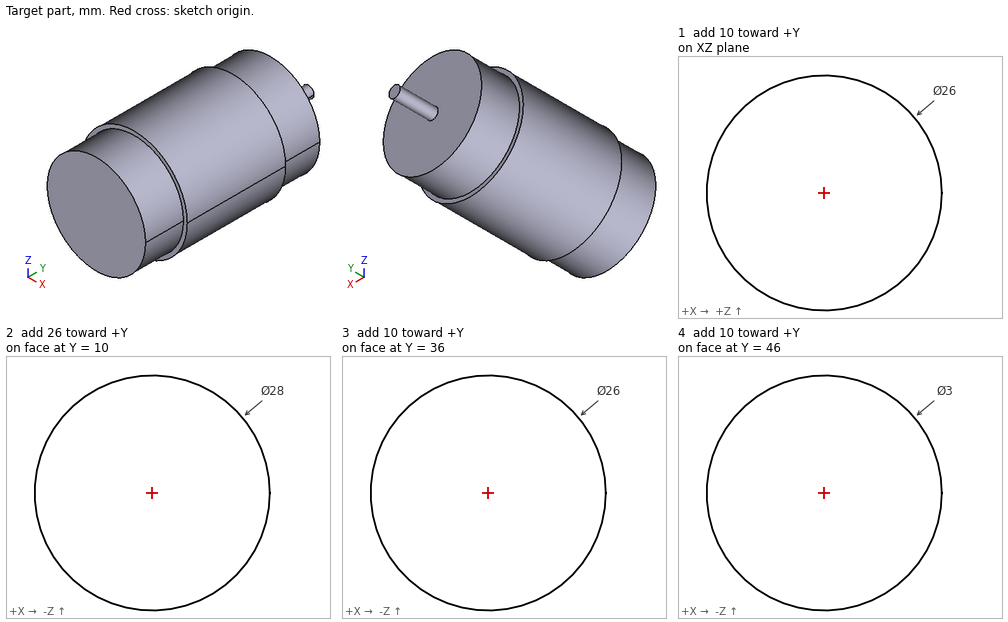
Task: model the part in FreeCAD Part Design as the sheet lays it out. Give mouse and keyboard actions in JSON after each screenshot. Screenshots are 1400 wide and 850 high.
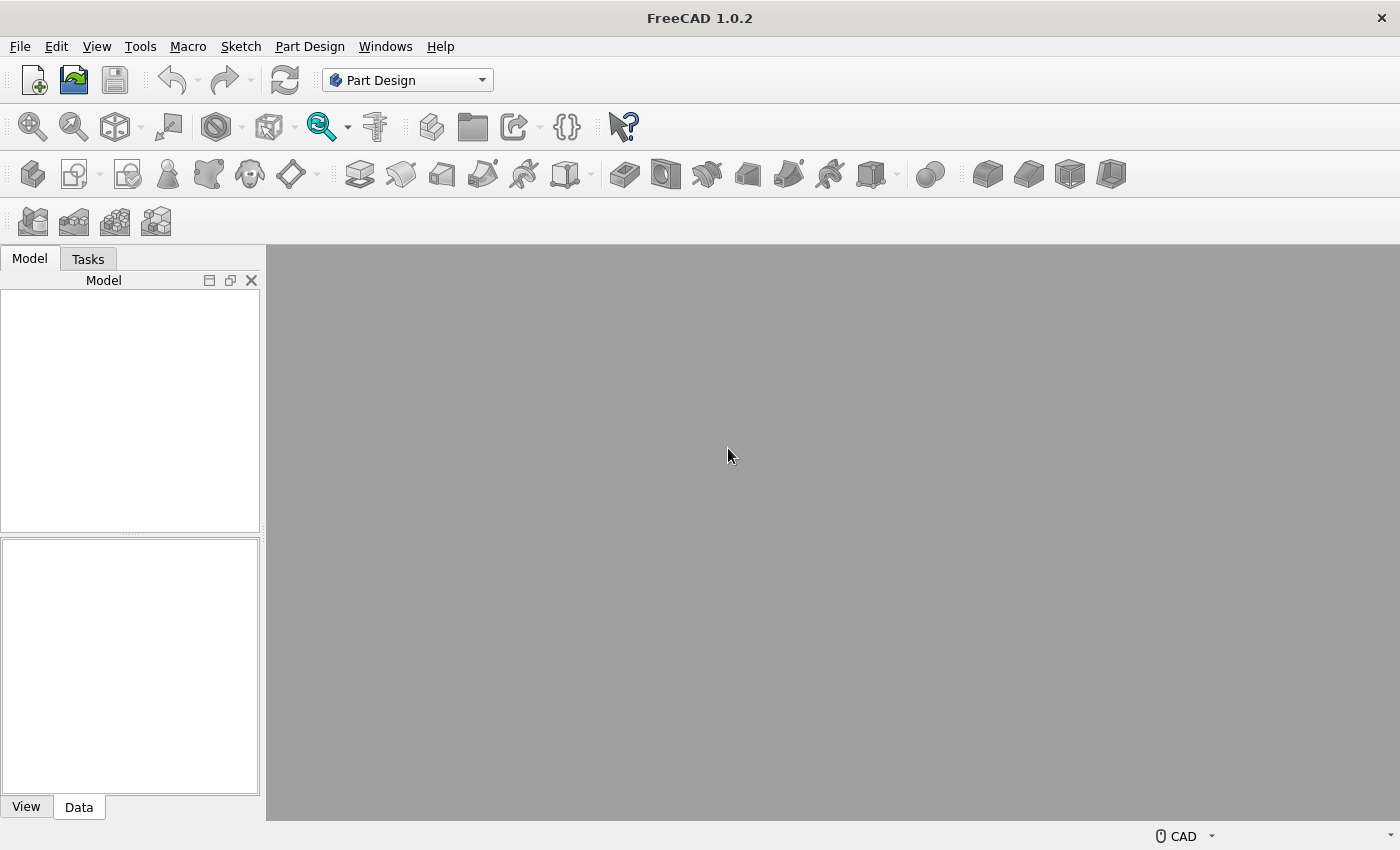
{"action": "left_click", "coordinate": [33, 80]}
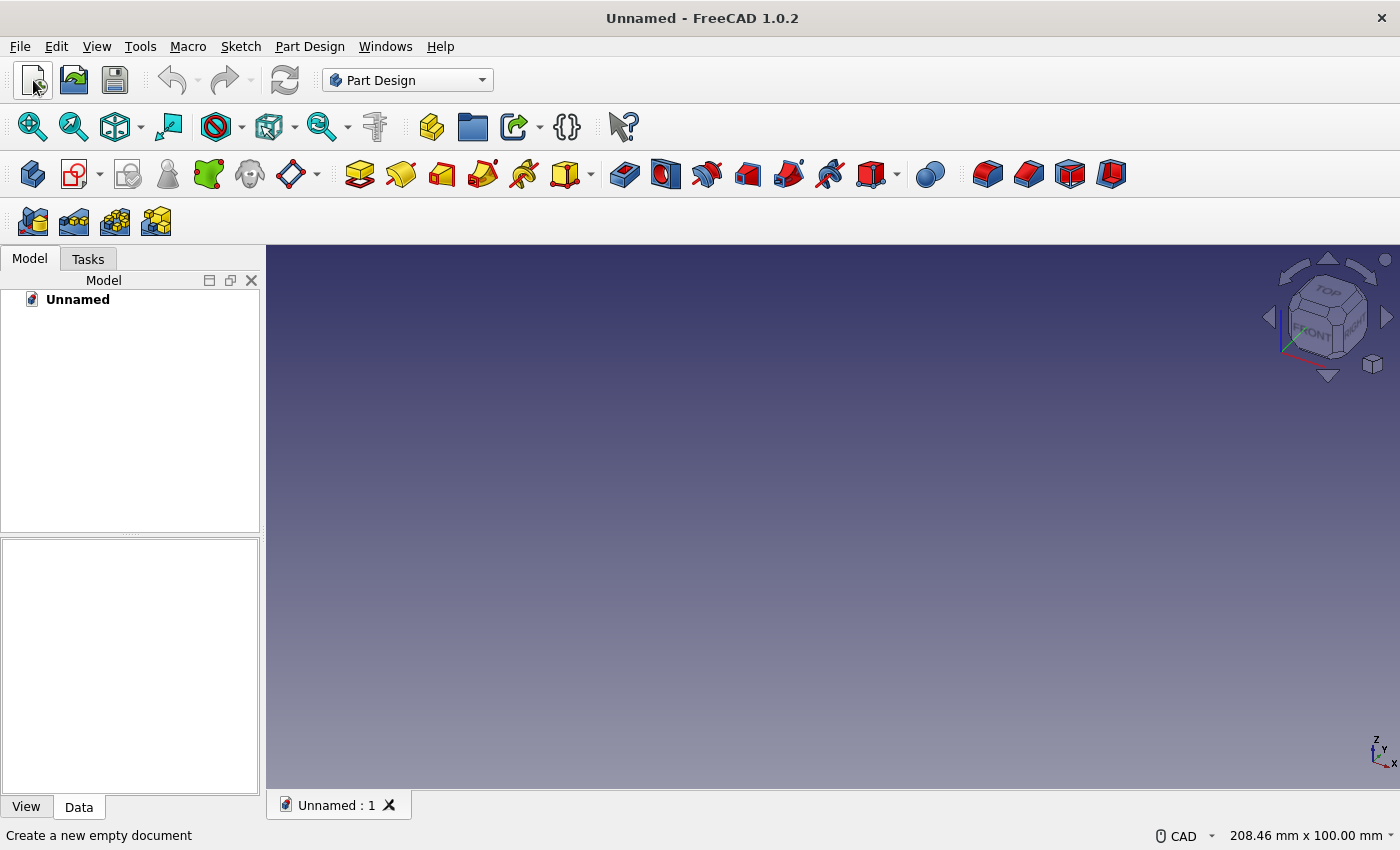
{"action": "left_click", "coordinate": [74, 174]}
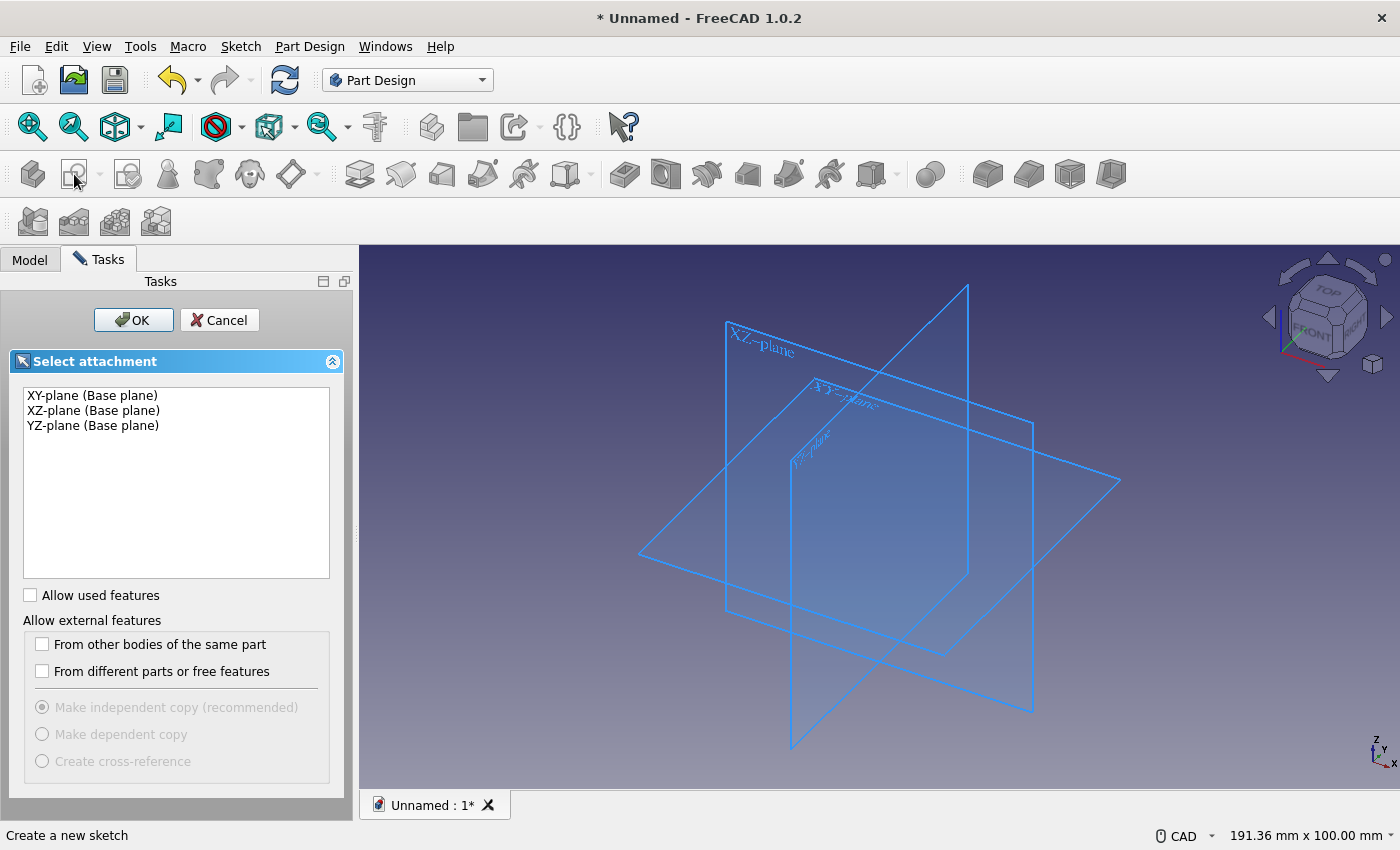
{"action": "left_click", "coordinate": [84, 410]}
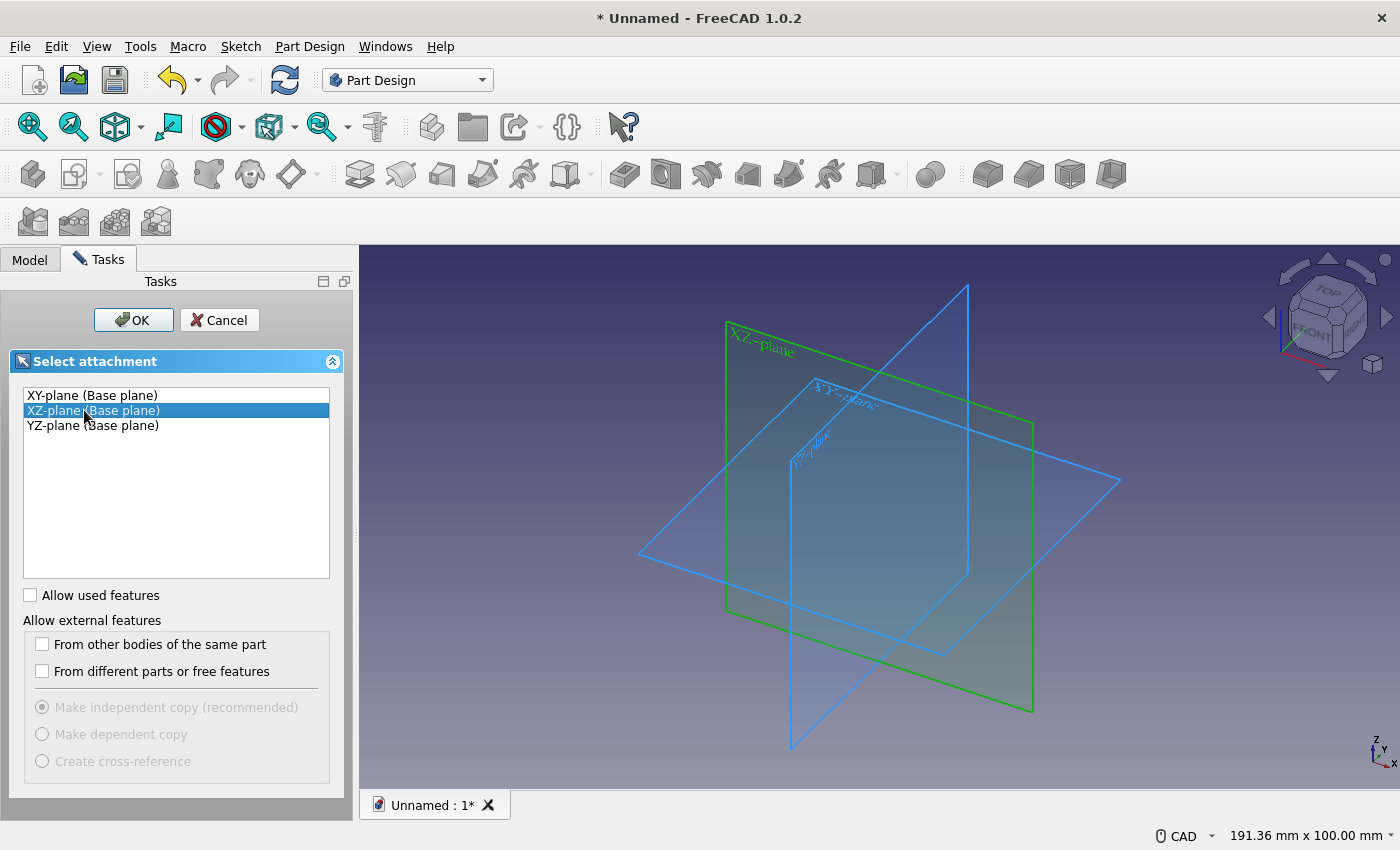
{"action": "left_click", "coordinate": [134, 320]}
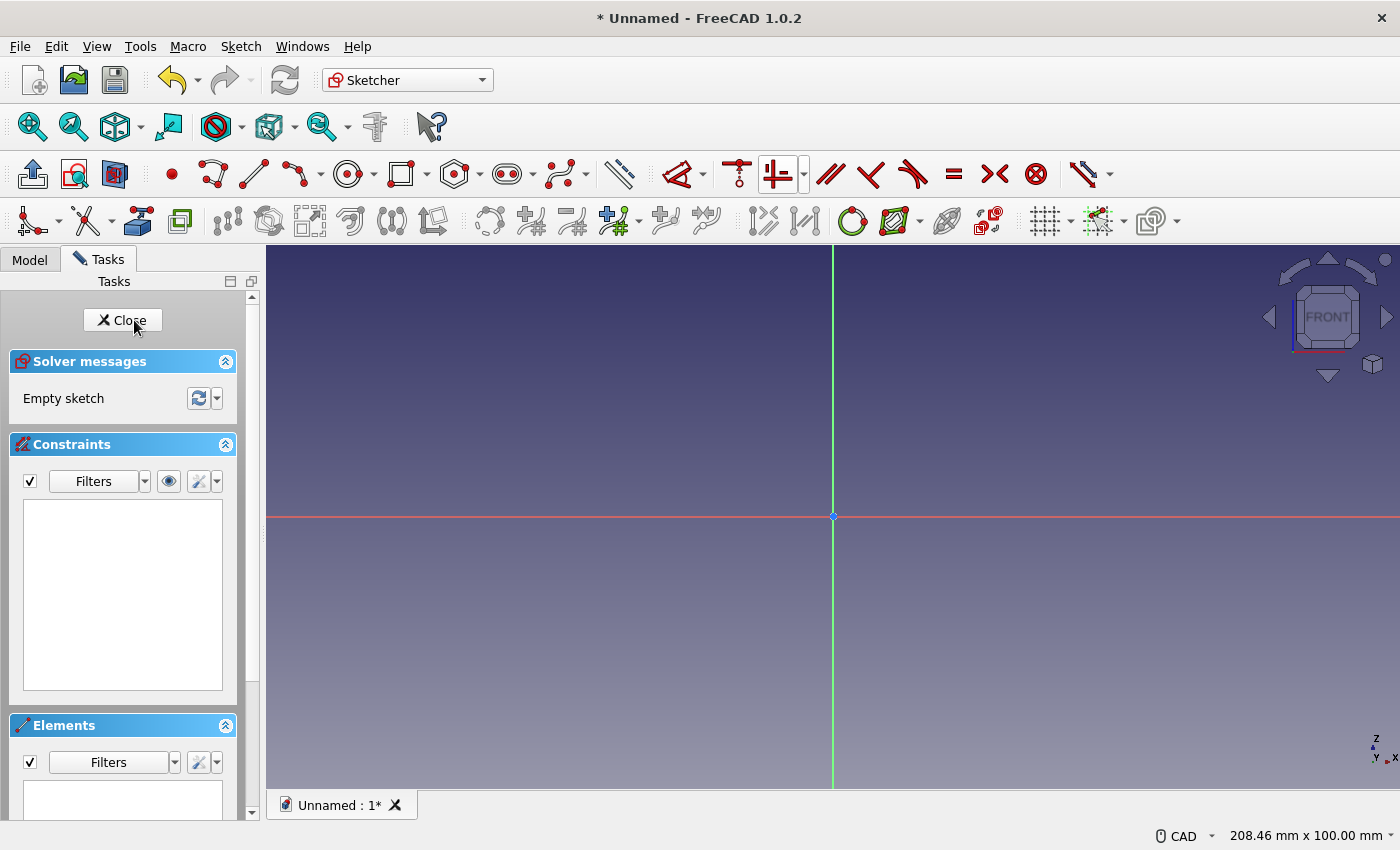
{"action": "scroll", "coordinate": [889, 517], "scroll_direction": "up", "scroll_amount": 4}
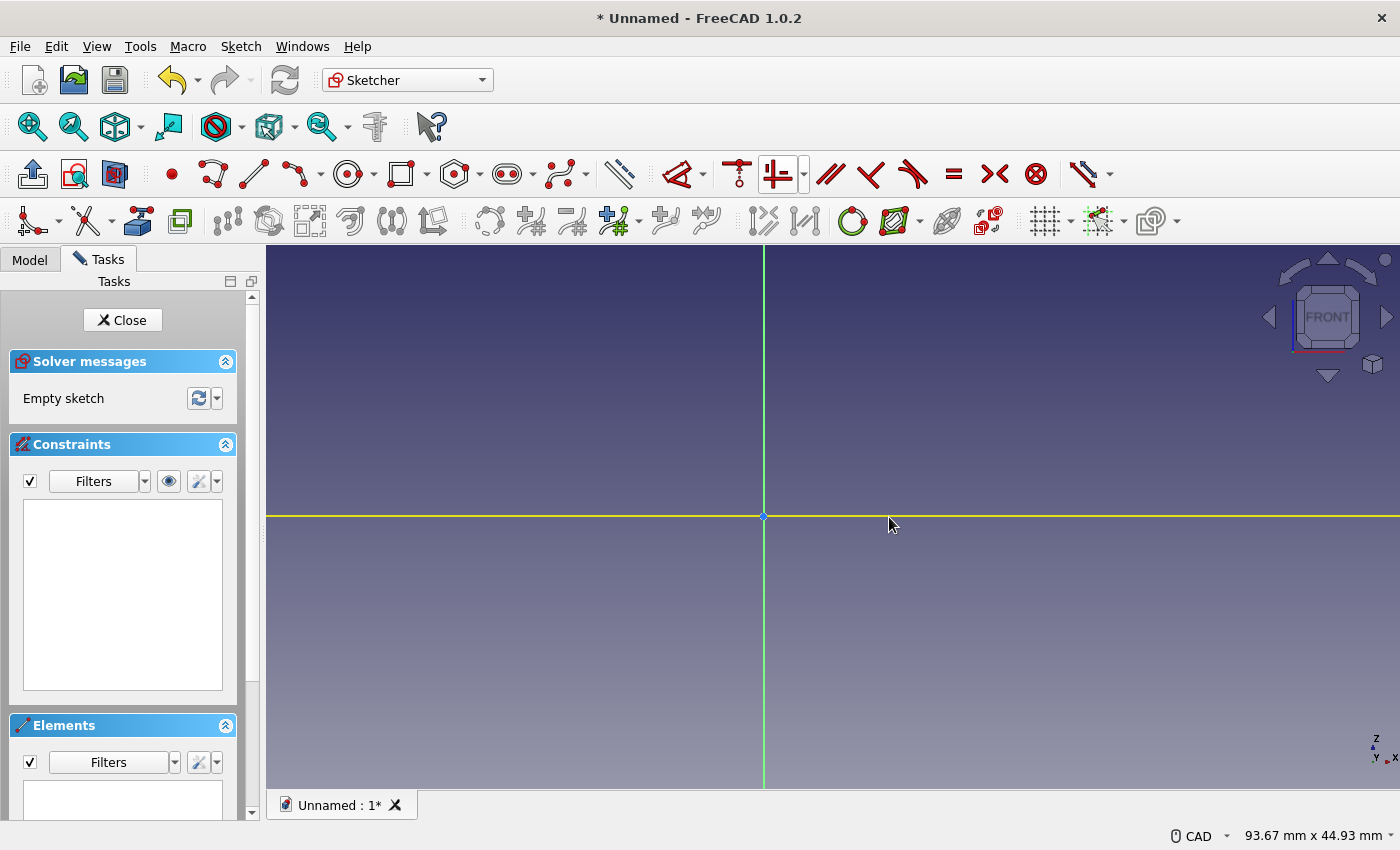
{"action": "left_click", "coordinate": [348, 174]}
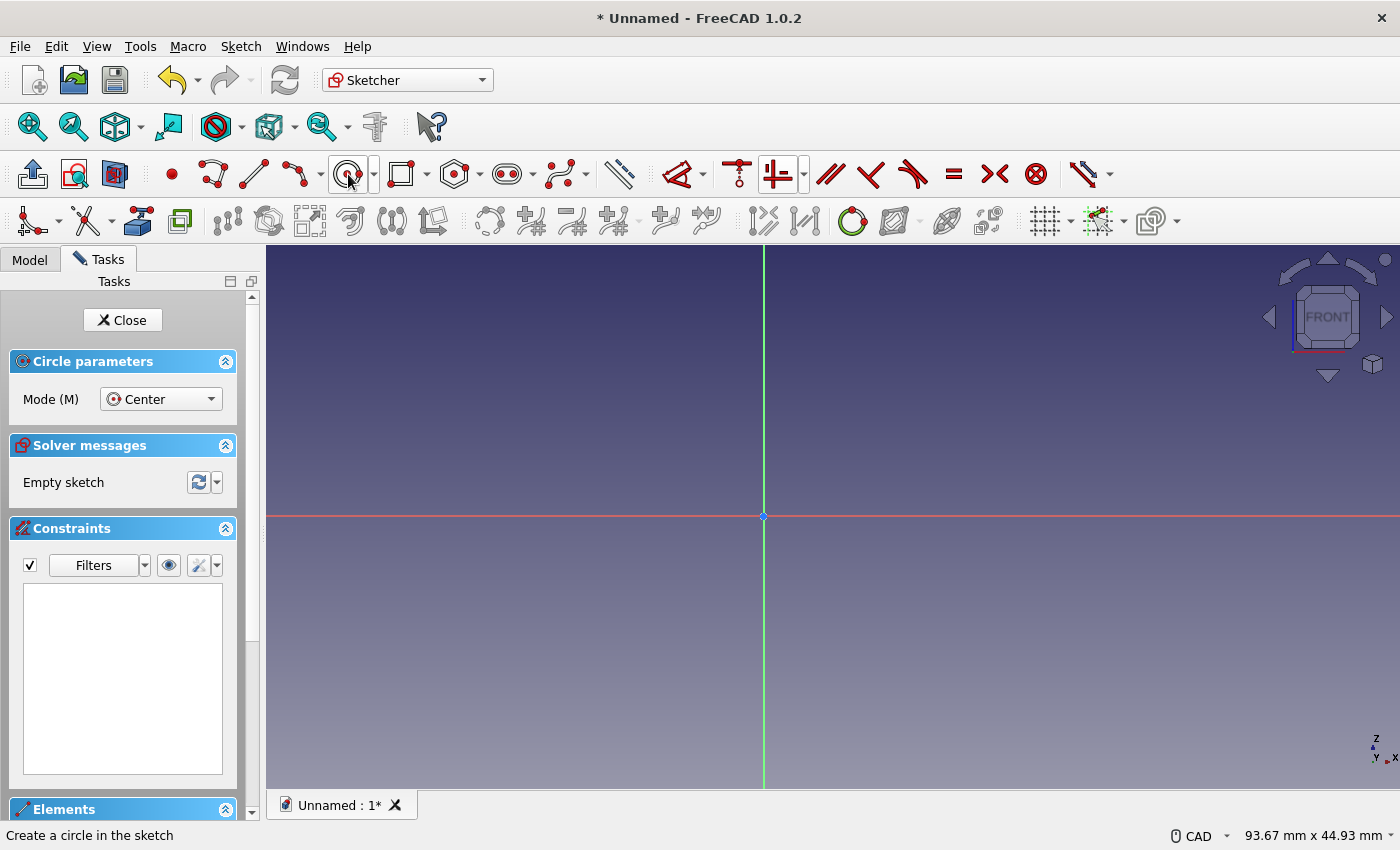
{"action": "left_click", "coordinate": [764, 516]}
{"action": "mouse_move", "coordinate": [875, 405]}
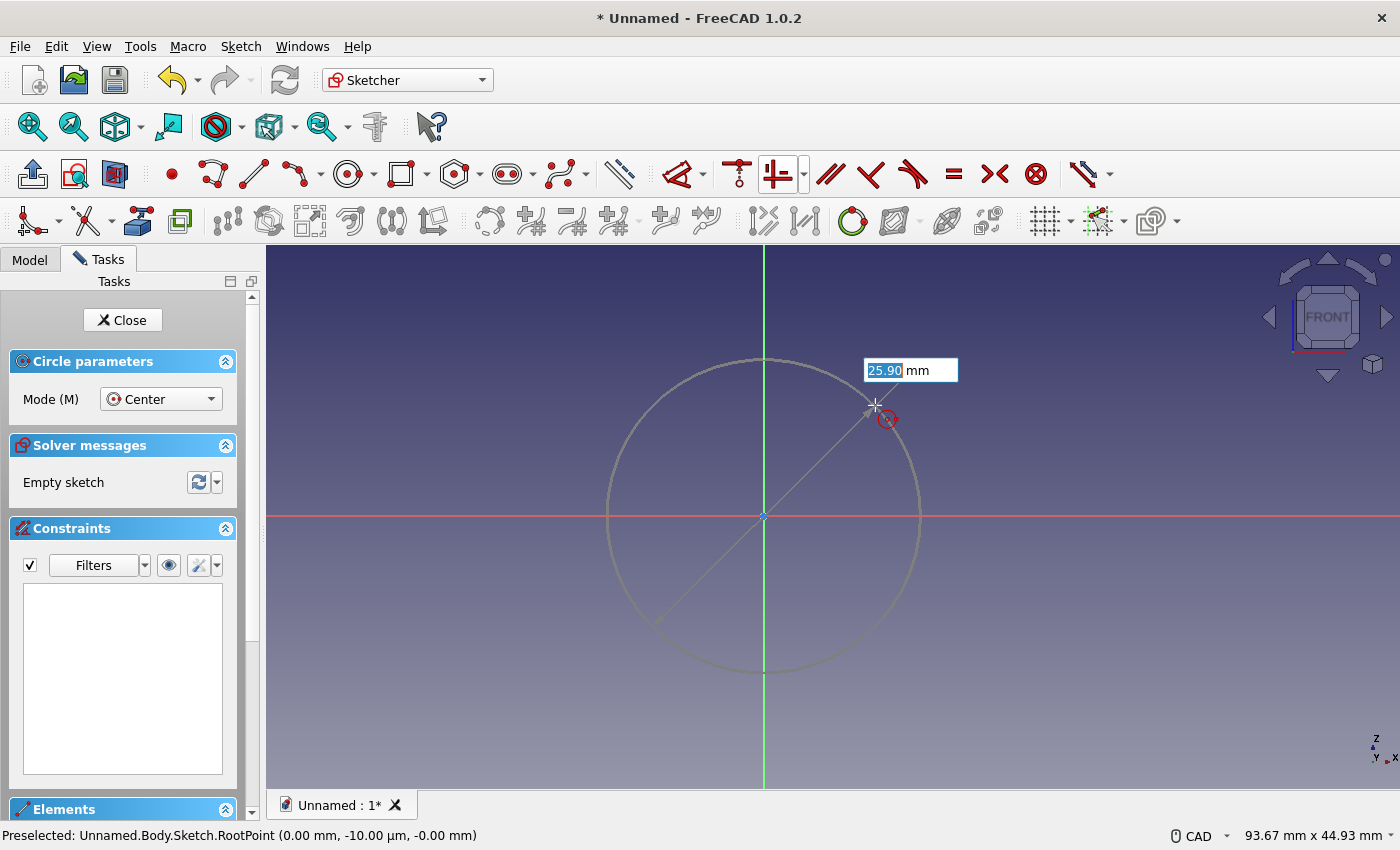
{"action": "type", "text": "26"}
{"action": "key", "text": "Return"}
{"action": "key", "text": "Escape"}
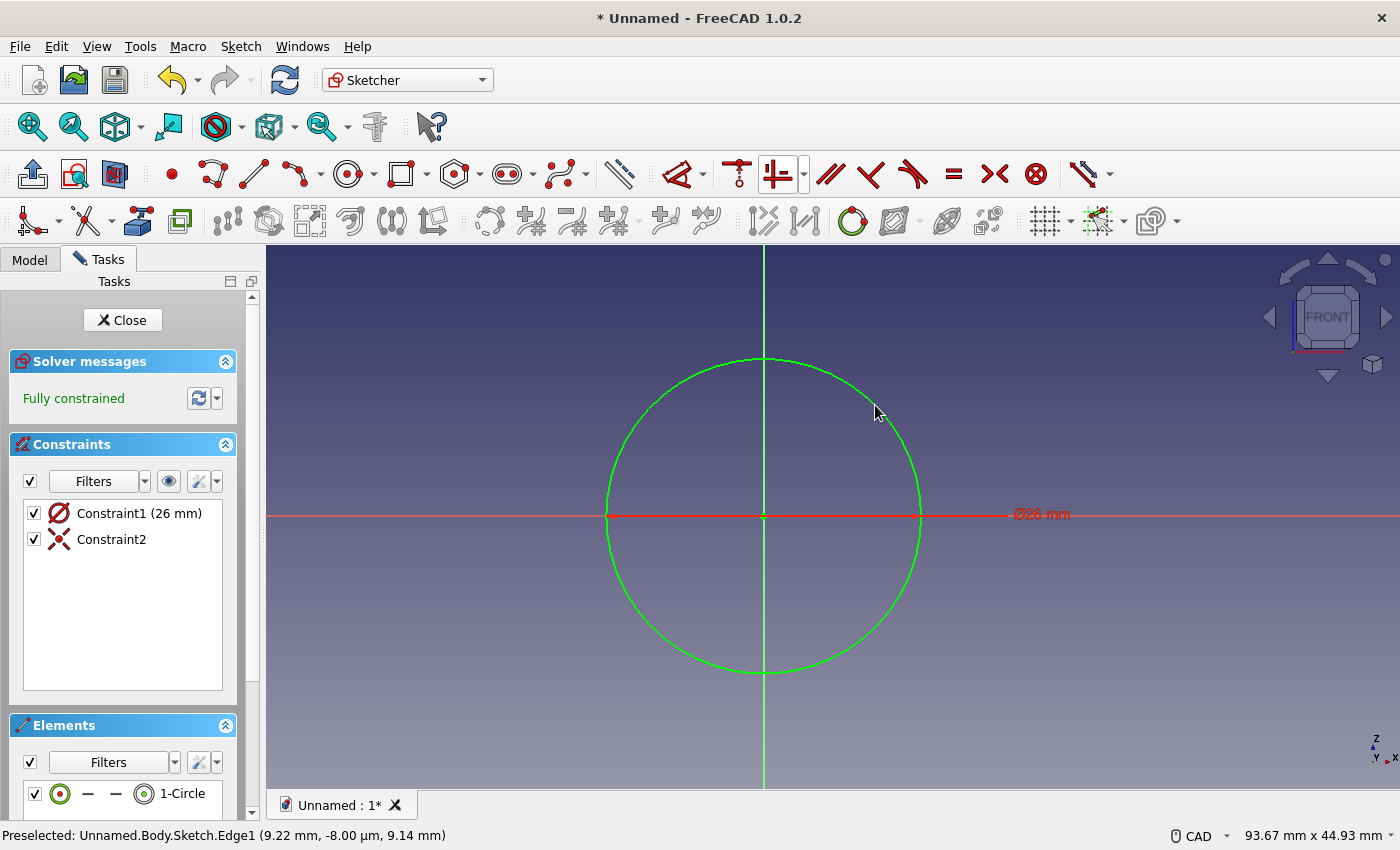
{"action": "left_click", "coordinate": [123, 320]}